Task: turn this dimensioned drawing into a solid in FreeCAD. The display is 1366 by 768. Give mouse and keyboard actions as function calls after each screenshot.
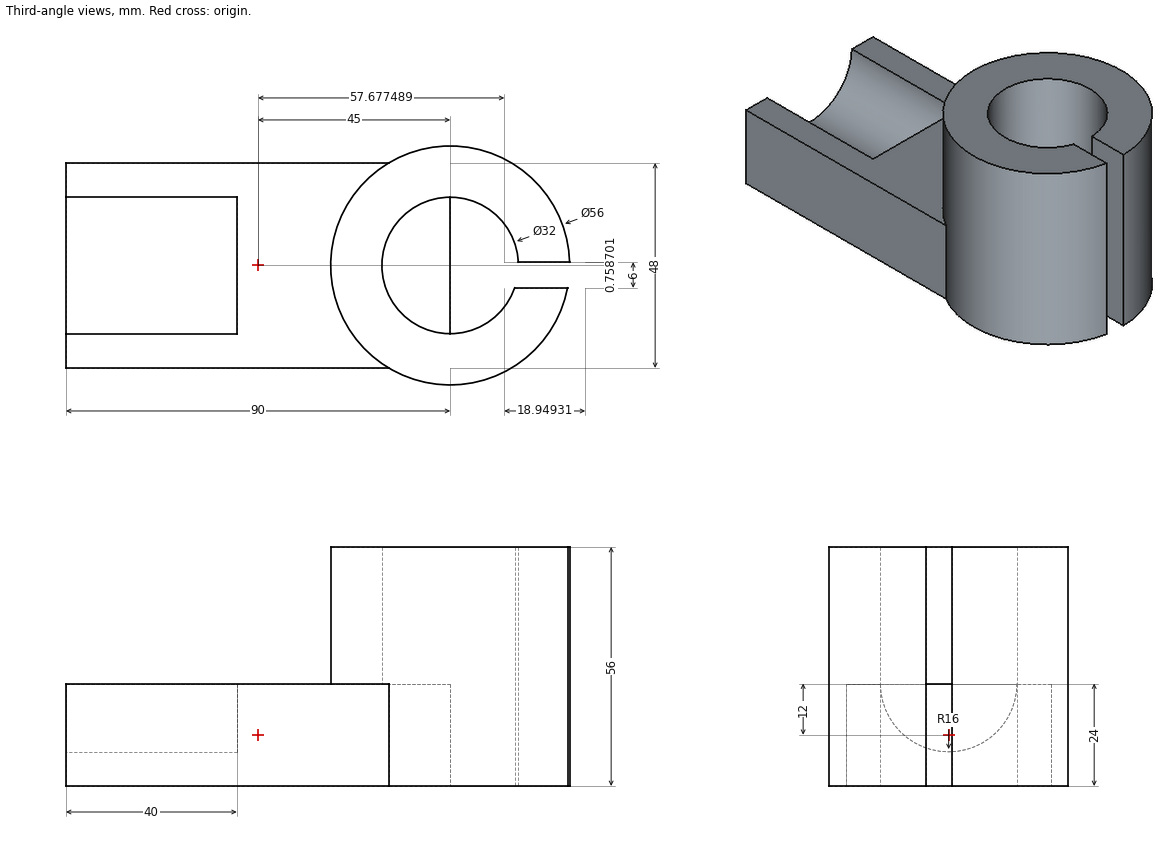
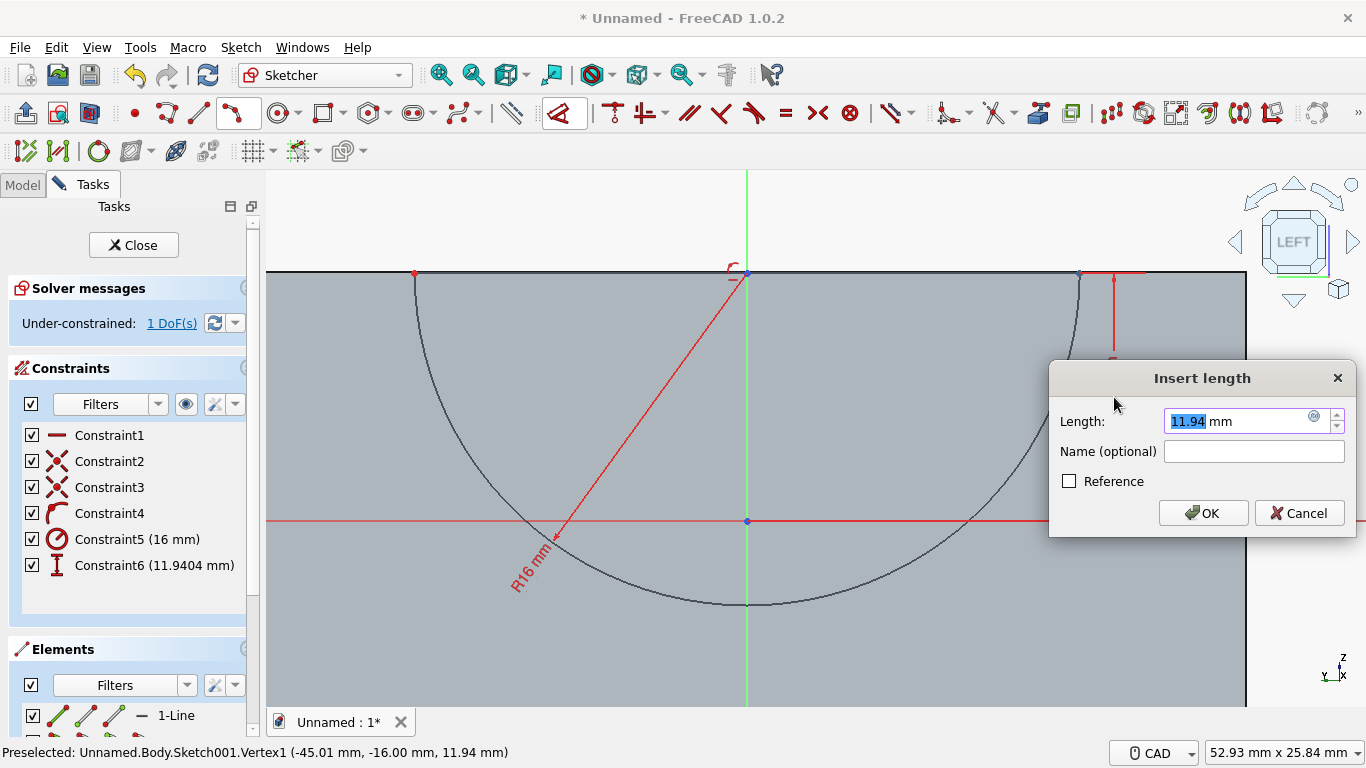
text(12)
key(Return)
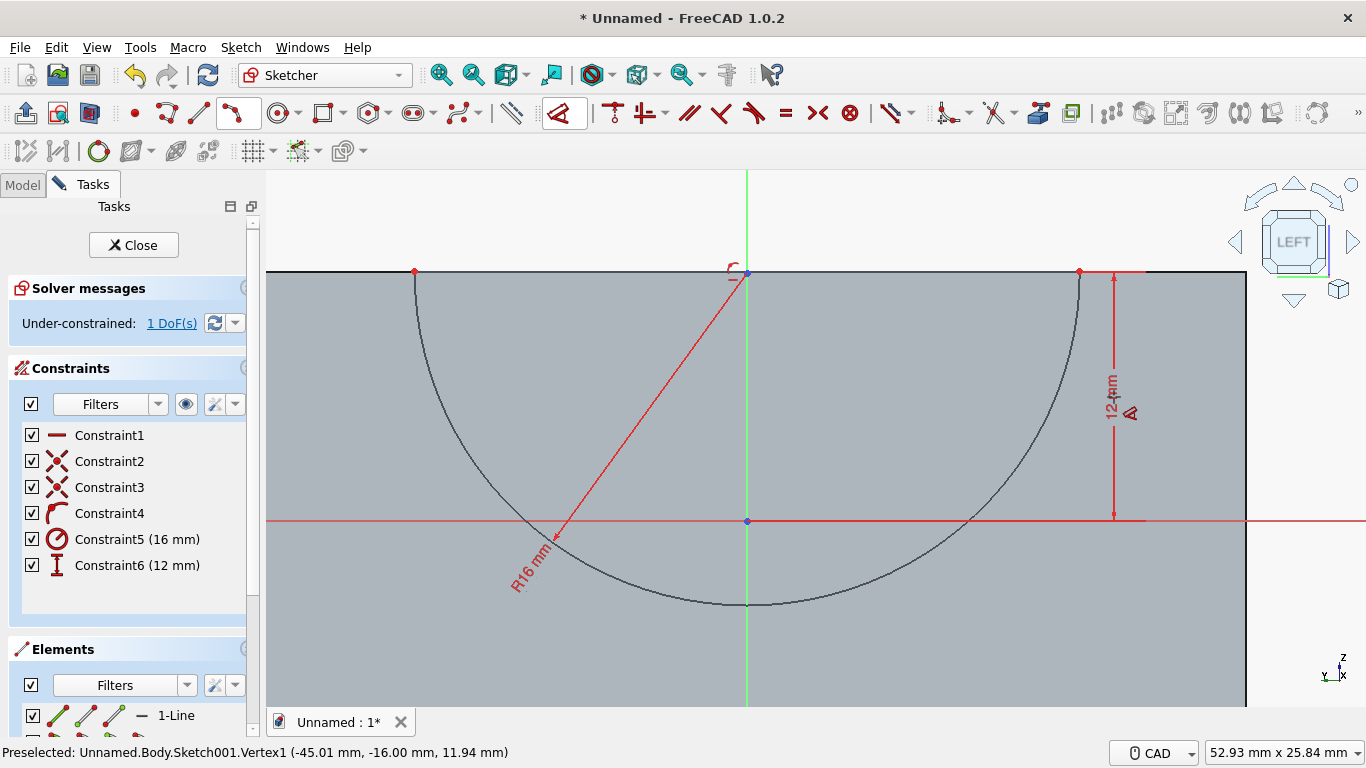
click(747, 273)
click(781, 397)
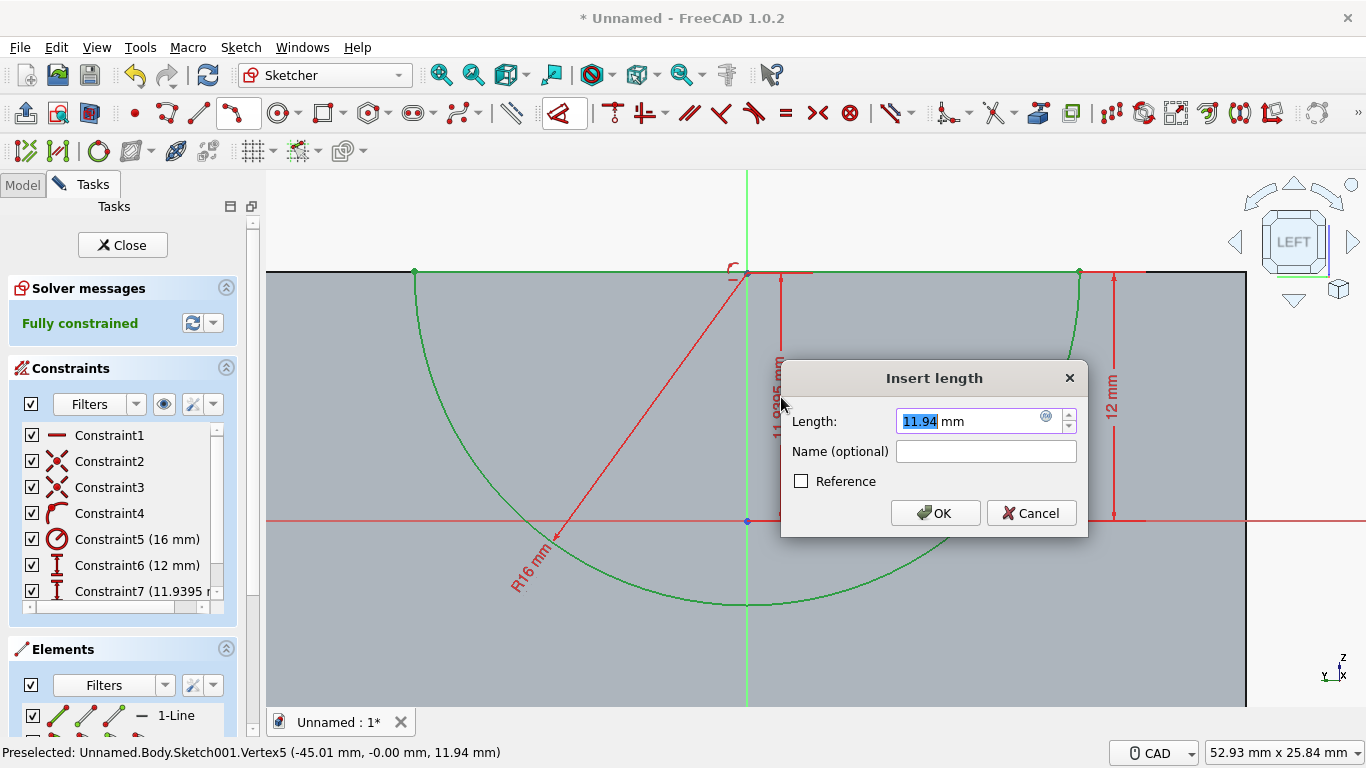
text(12)
key(Return)
key(Escape)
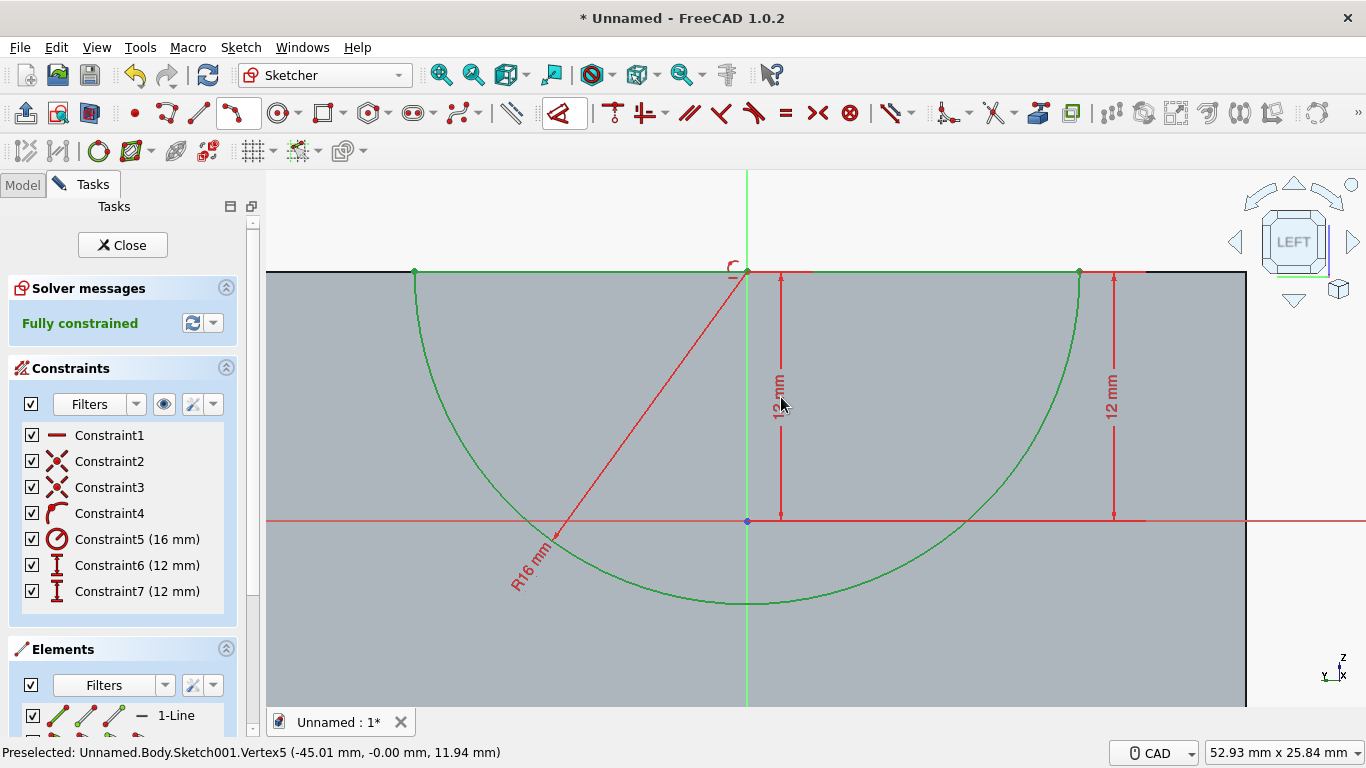
click(123, 245)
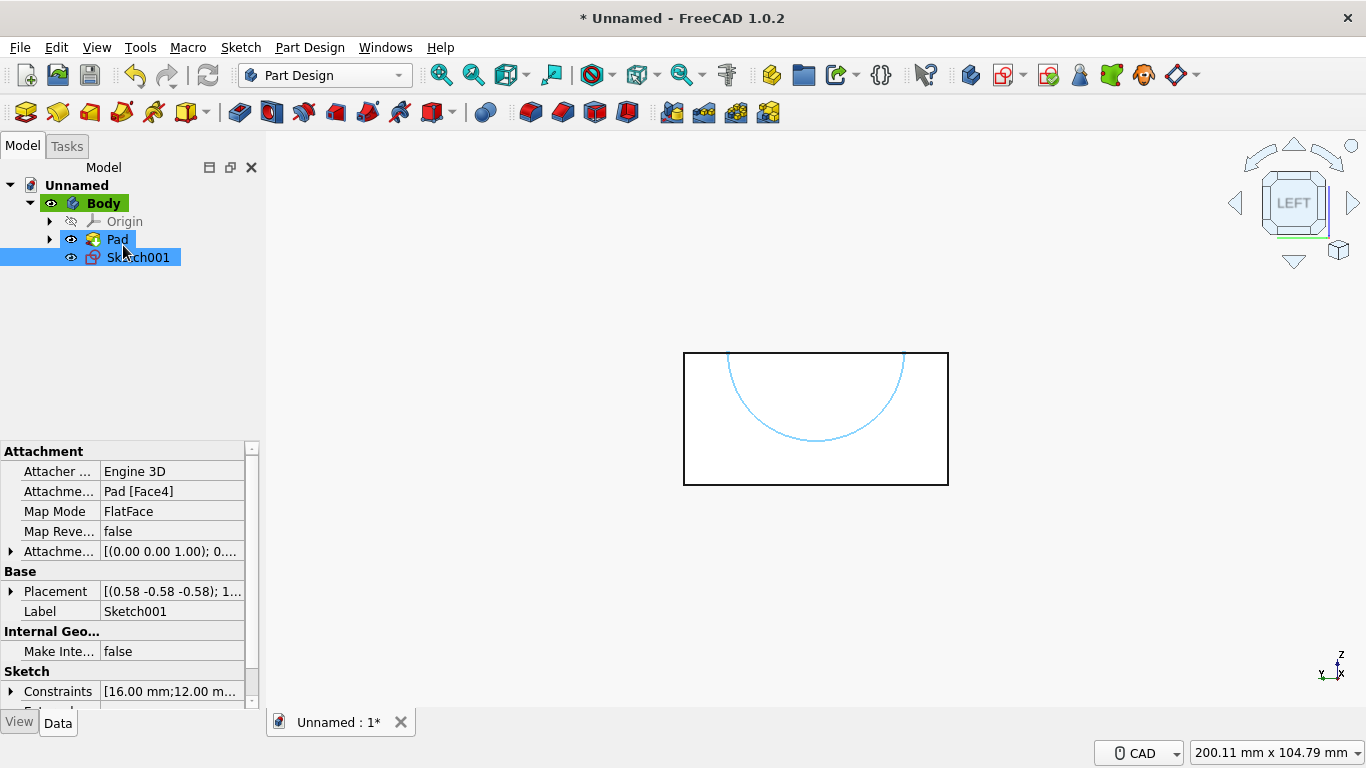
click(240, 112)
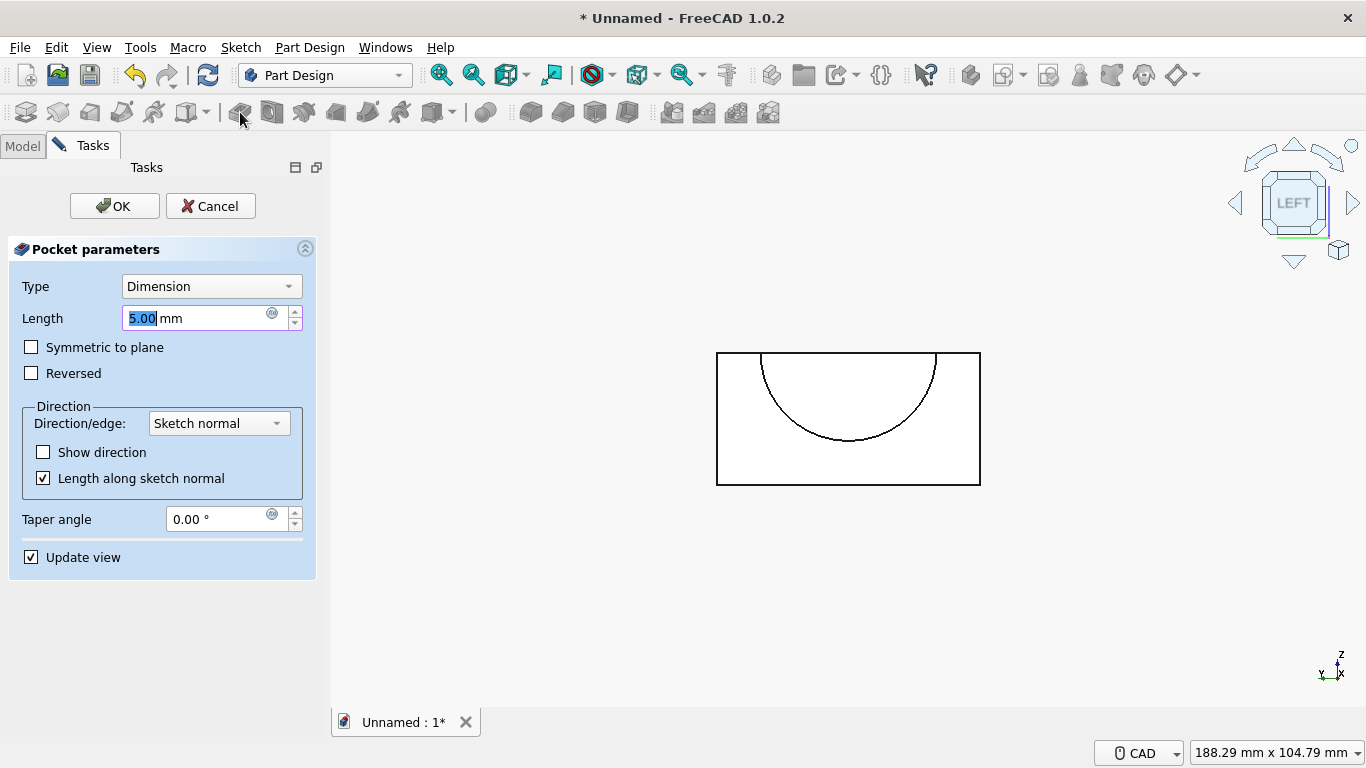
text(40)
key(Tab)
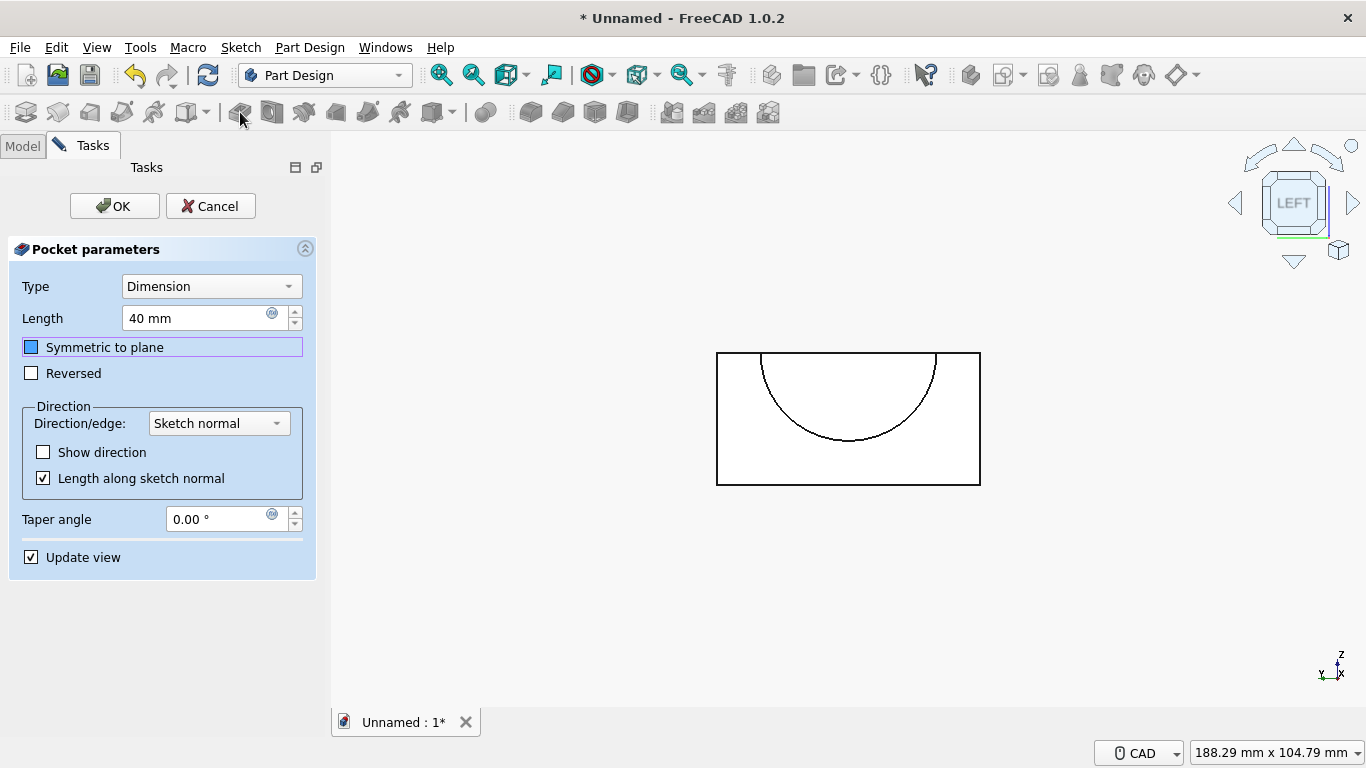
click(115, 206)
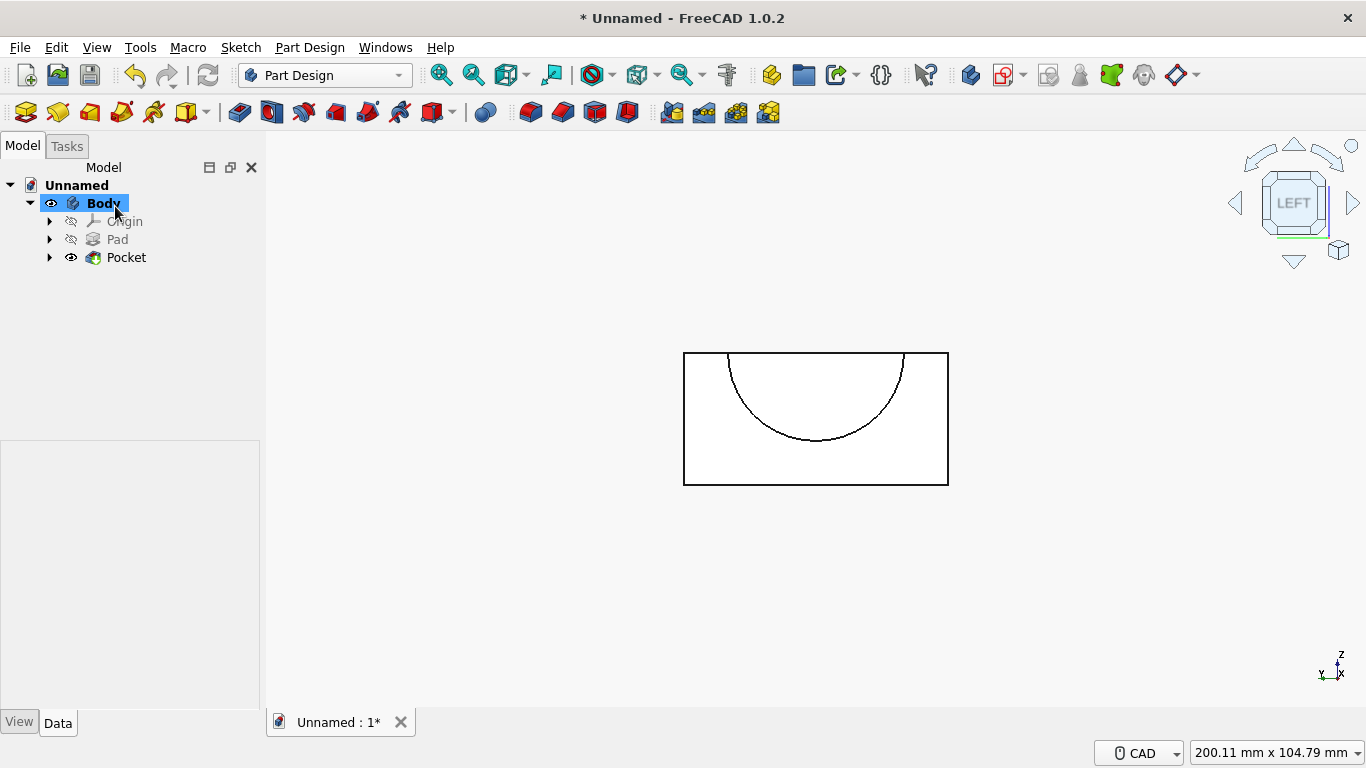
key(v)
key(f)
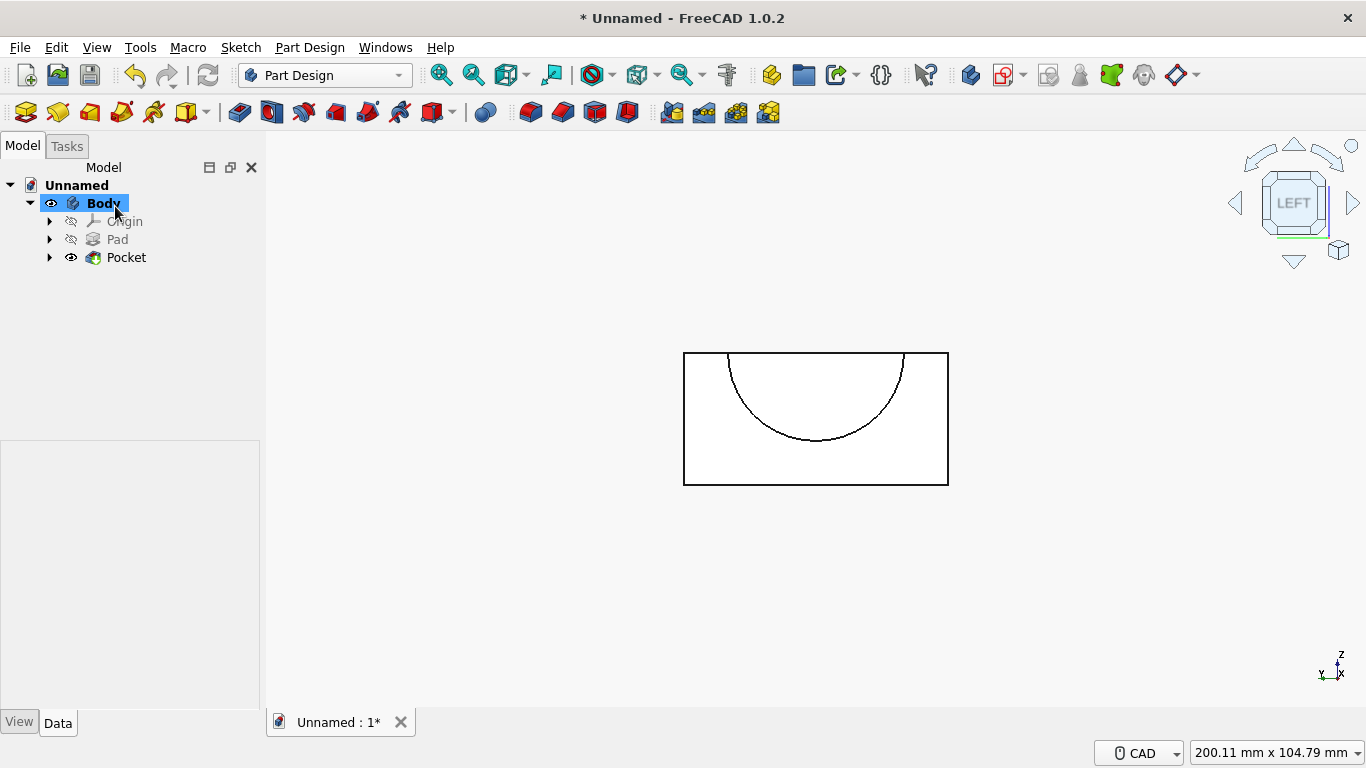
key(5)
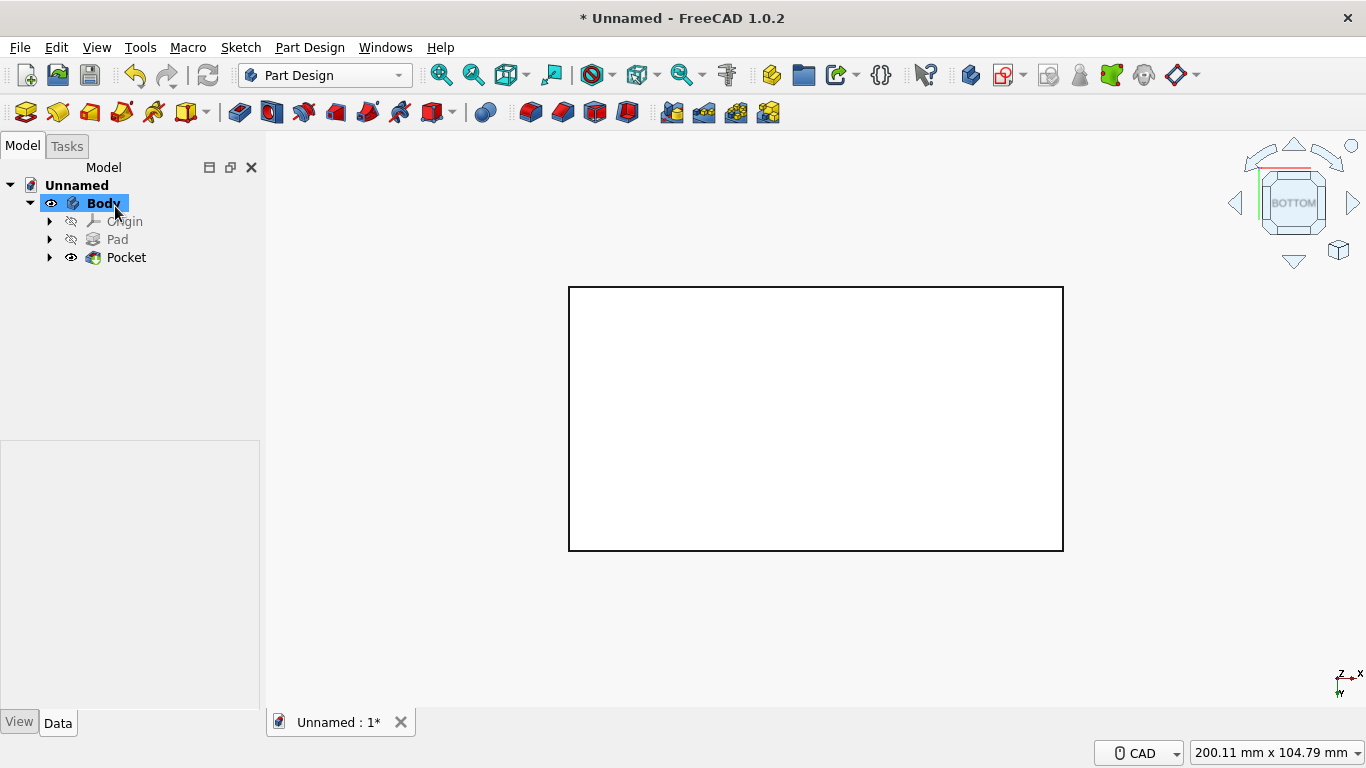
click(887, 418)